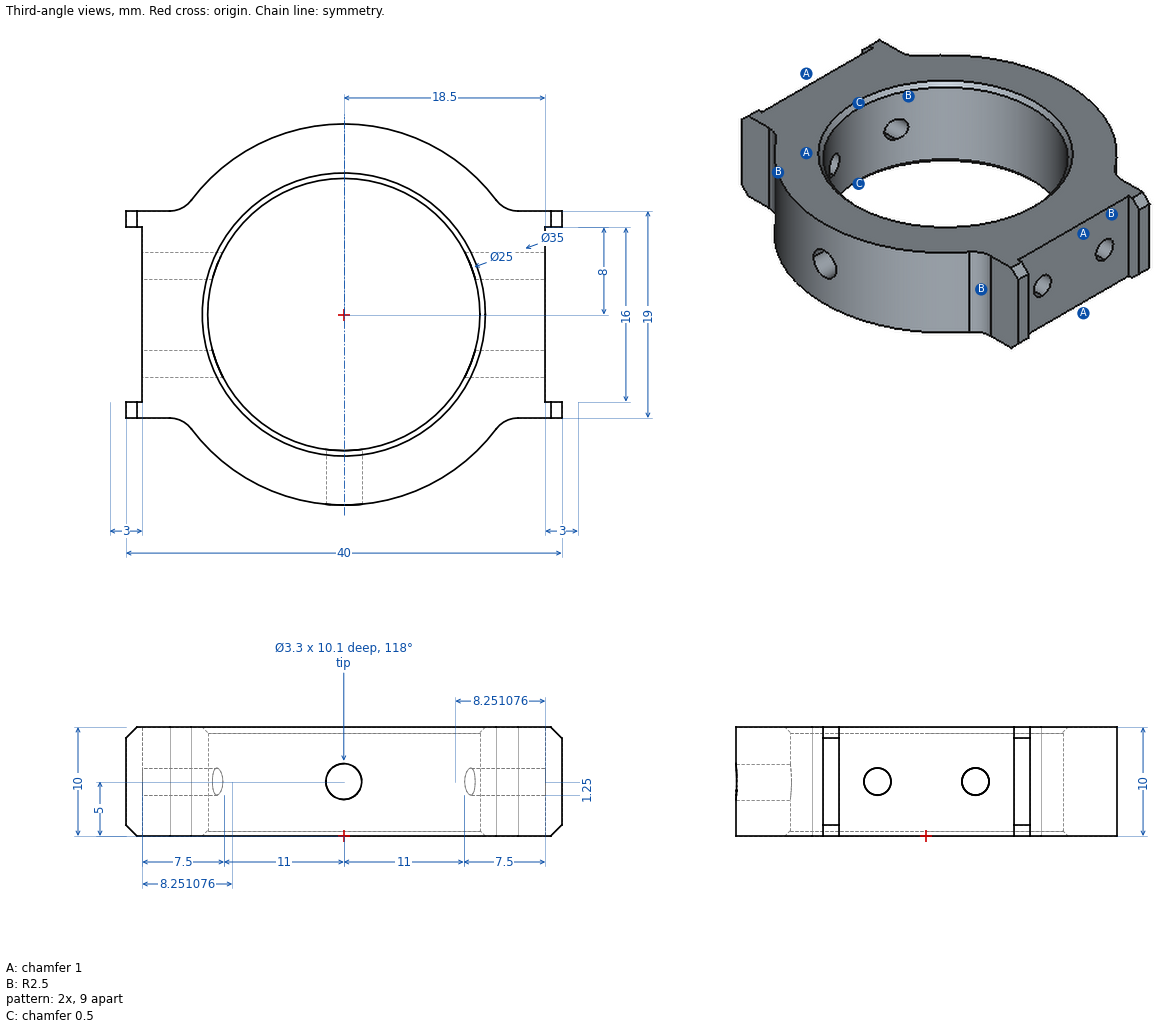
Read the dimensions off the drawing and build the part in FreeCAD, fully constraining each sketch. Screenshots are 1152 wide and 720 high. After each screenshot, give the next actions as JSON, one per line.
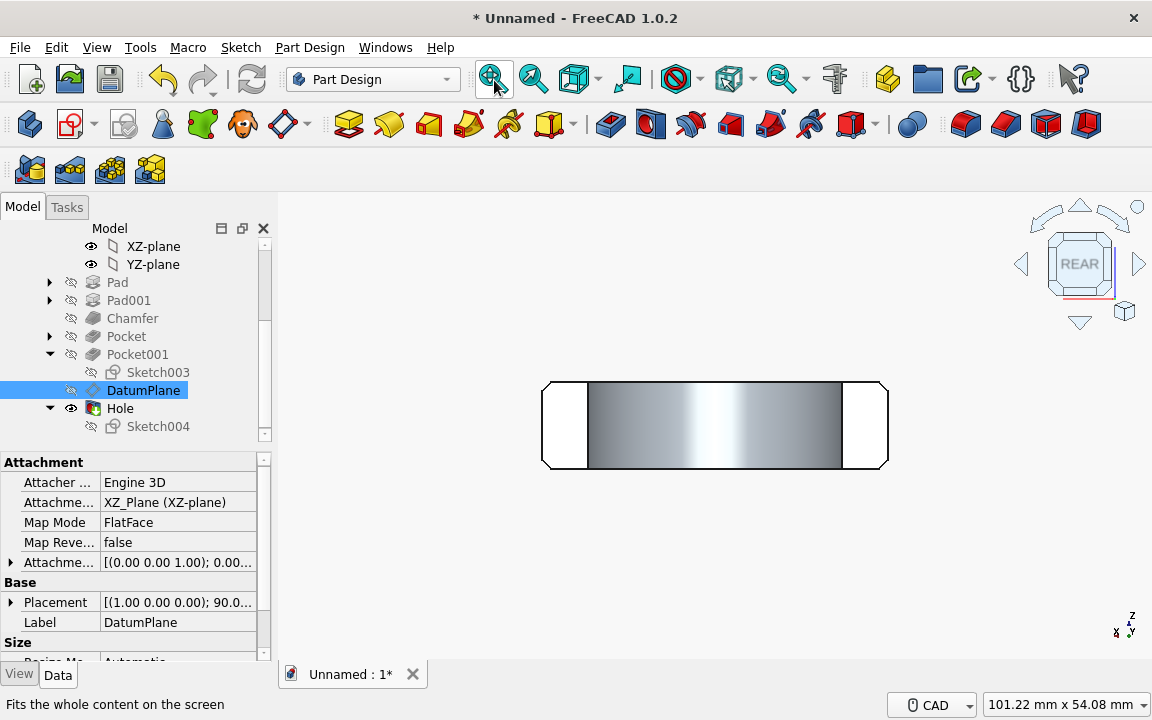
{"action": "left_click", "coordinate": [494, 80]}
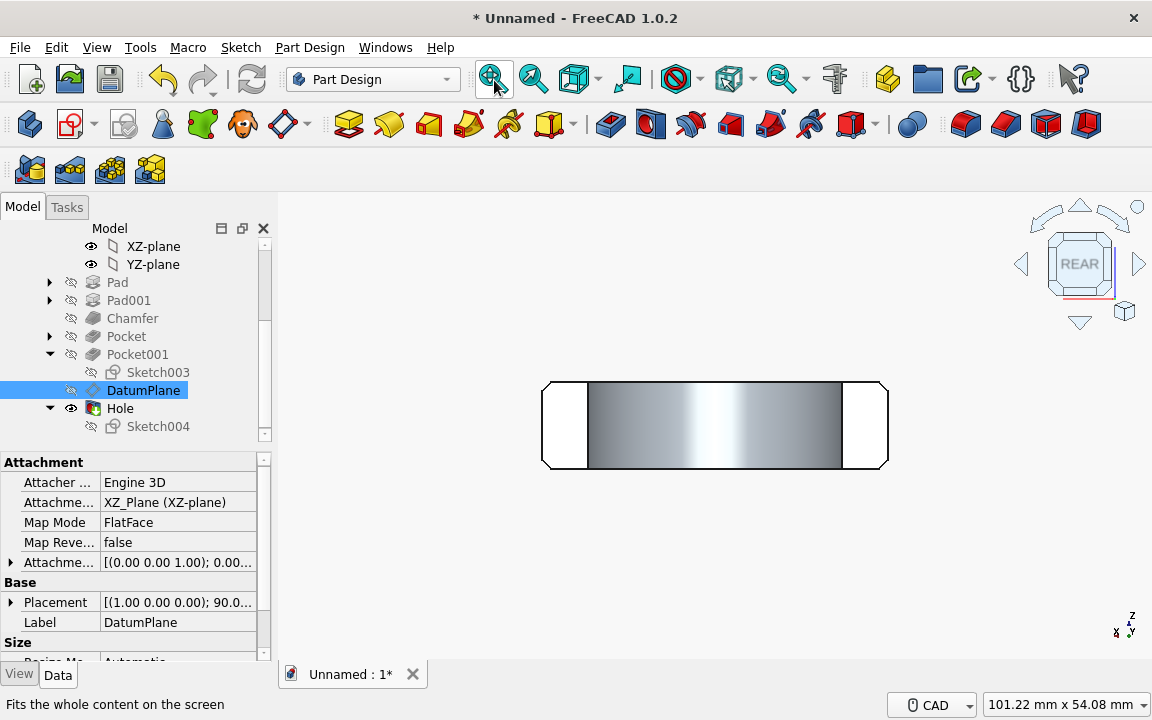
{"action": "key", "text": "6"}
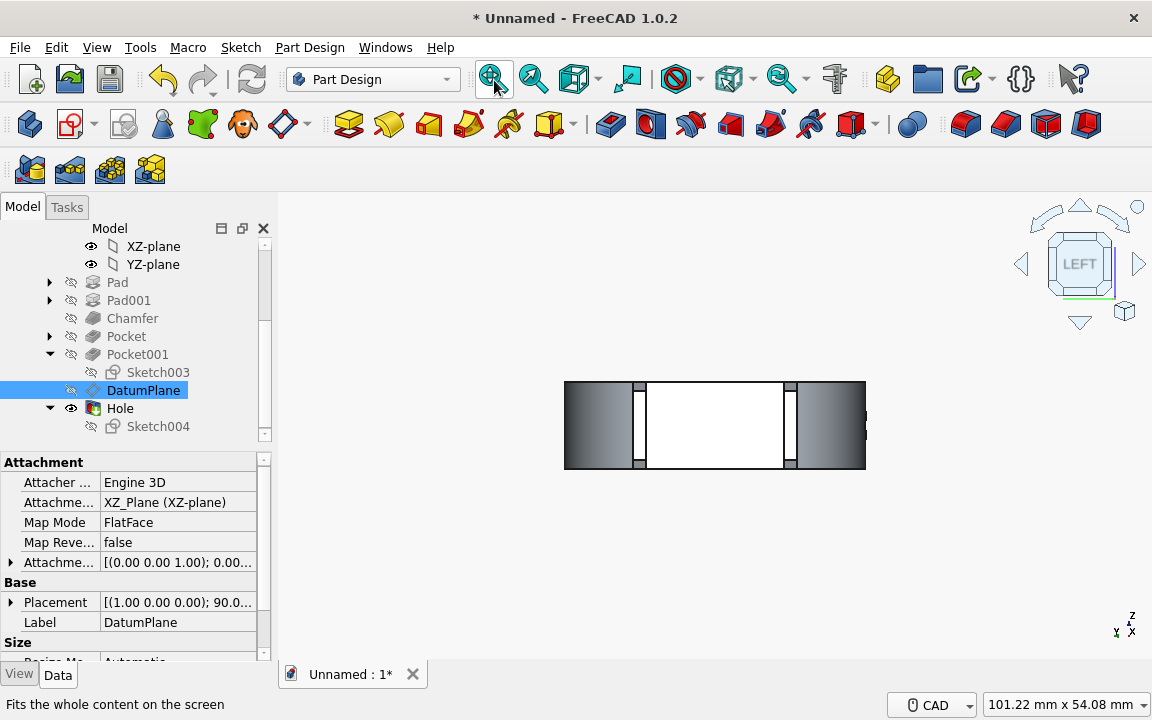
{"action": "left_click", "coordinate": [494, 80]}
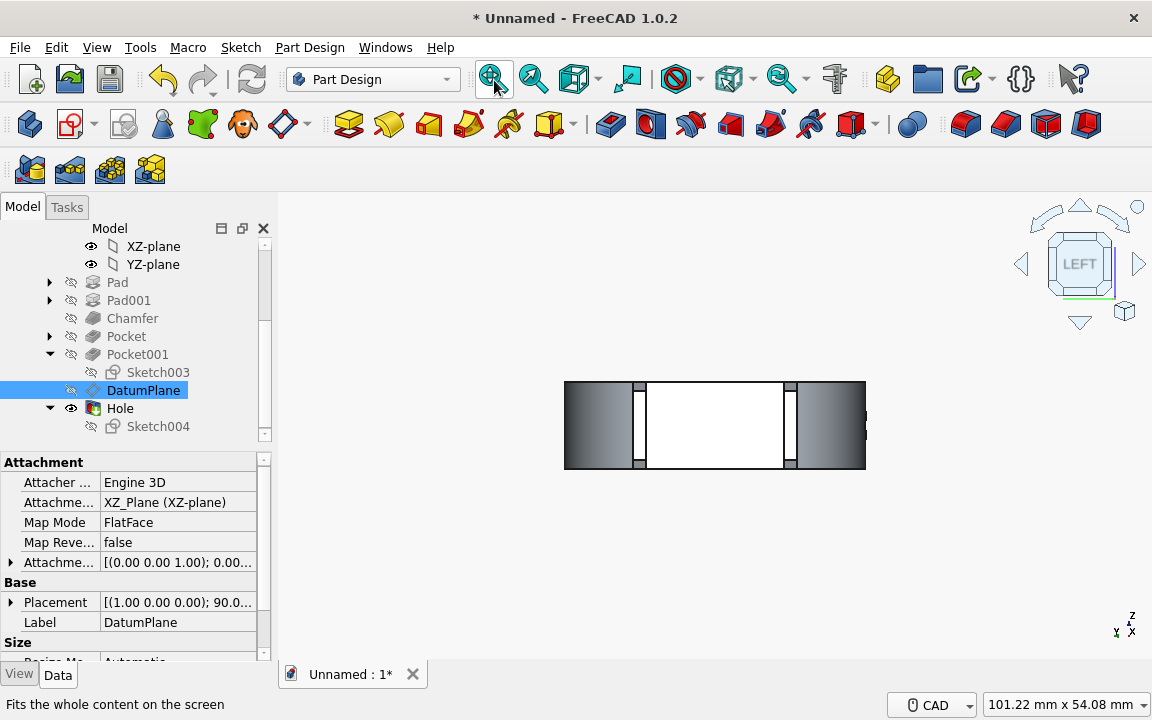
{"action": "key", "text": "v 3"}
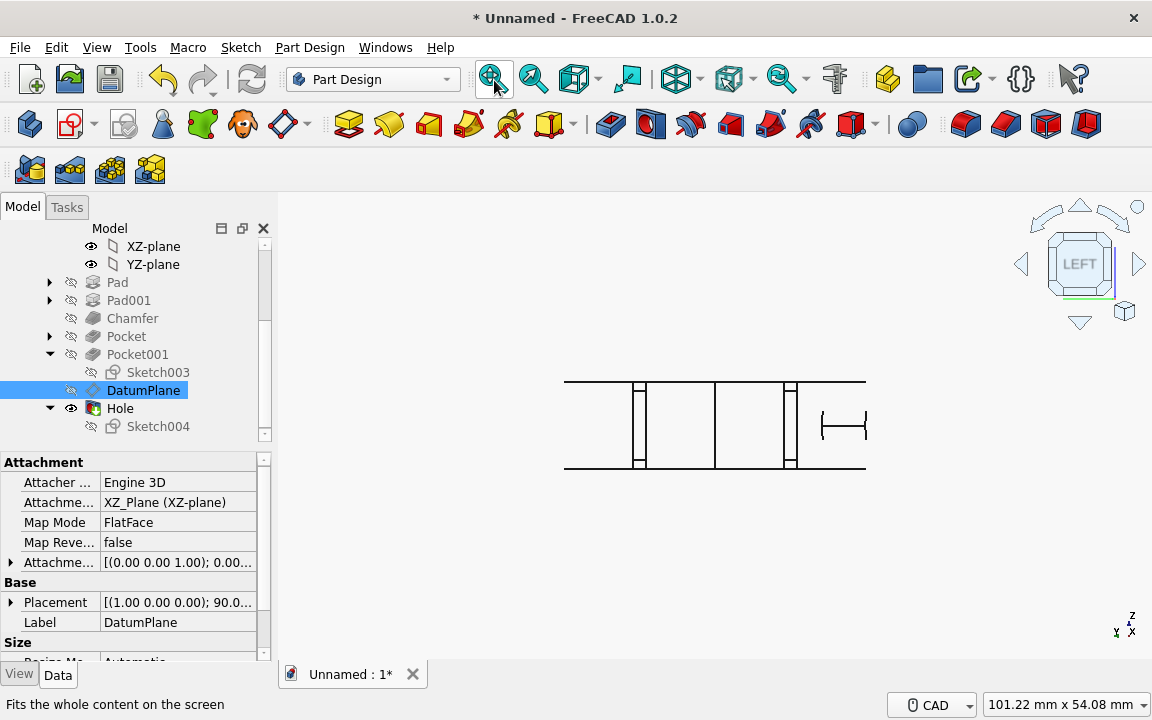
{"action": "key", "text": "0"}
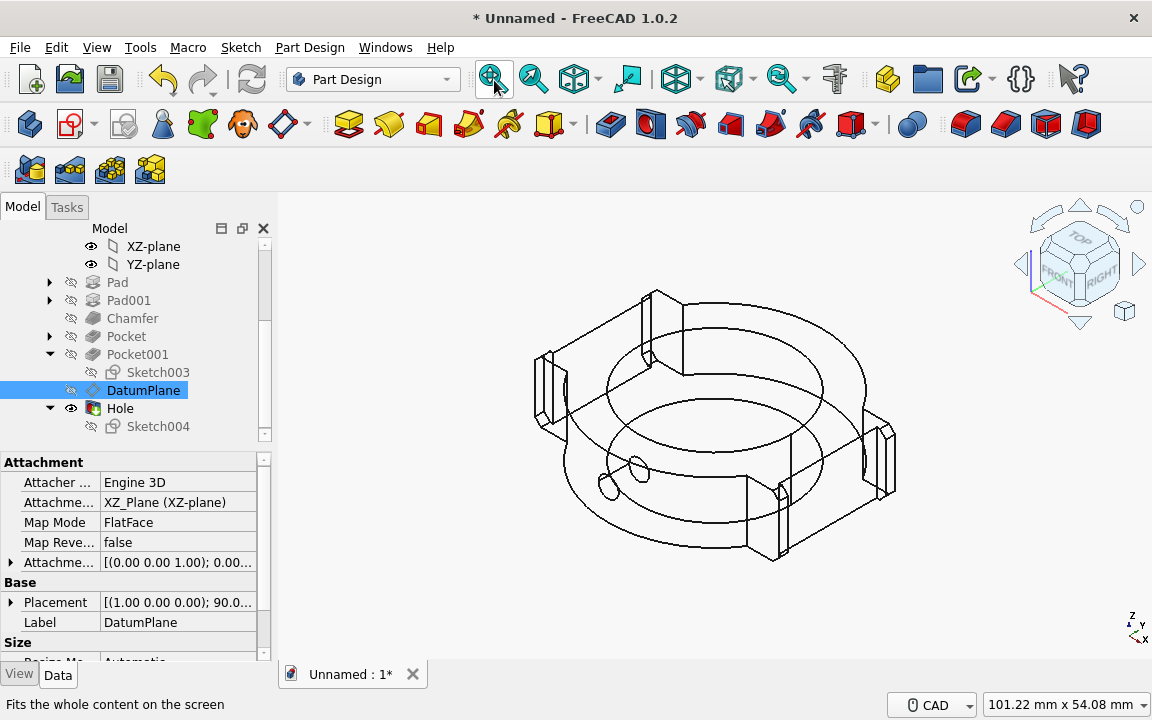
{"action": "left_click", "coordinate": [567, 427]}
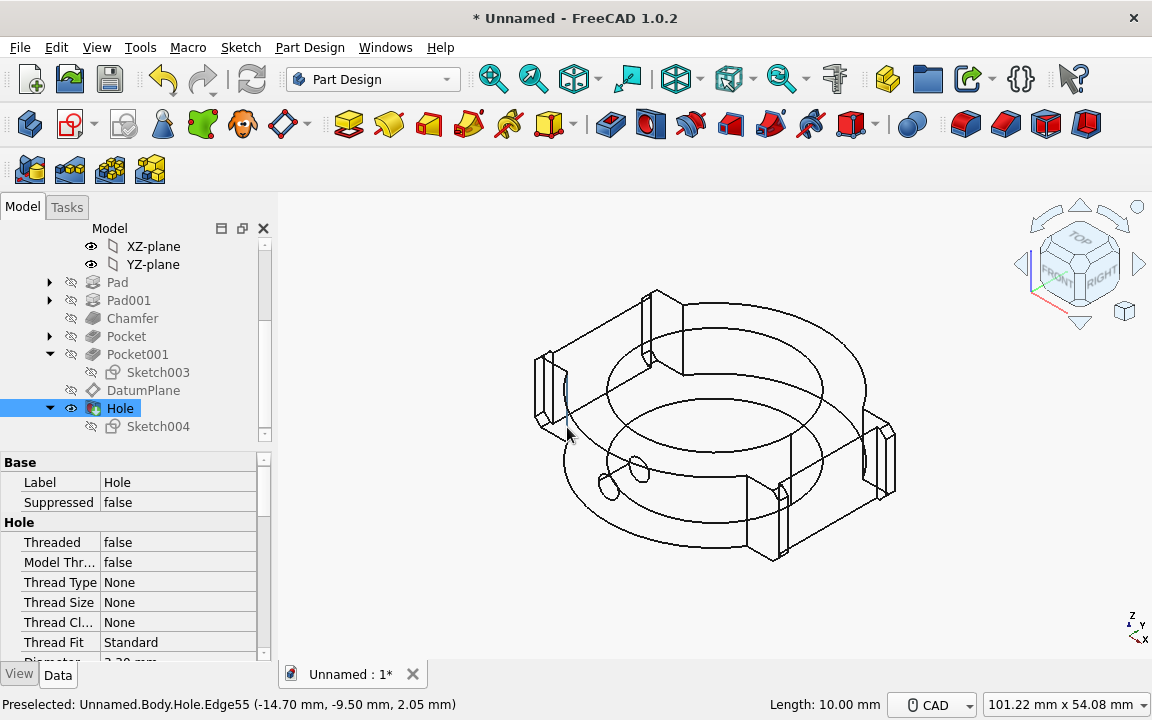
{"action": "left_click", "coordinate": [747, 510], "text": "ctrl"}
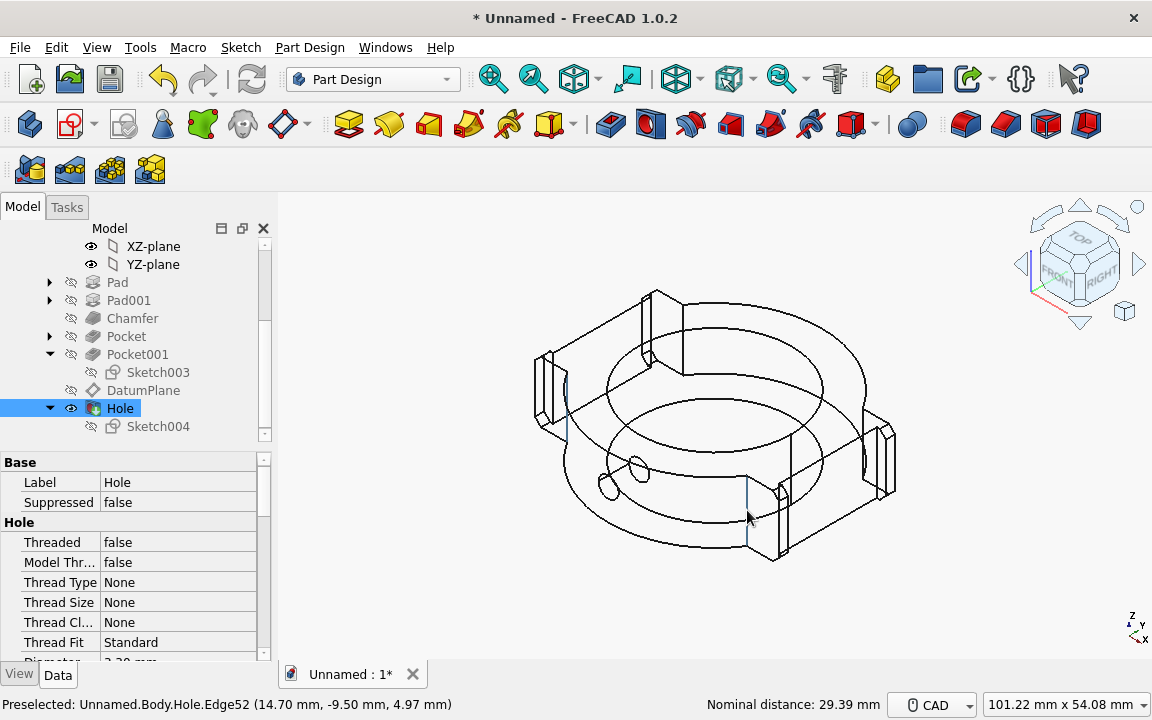
{"action": "left_click", "coordinate": [863, 443], "text": "ctrl"}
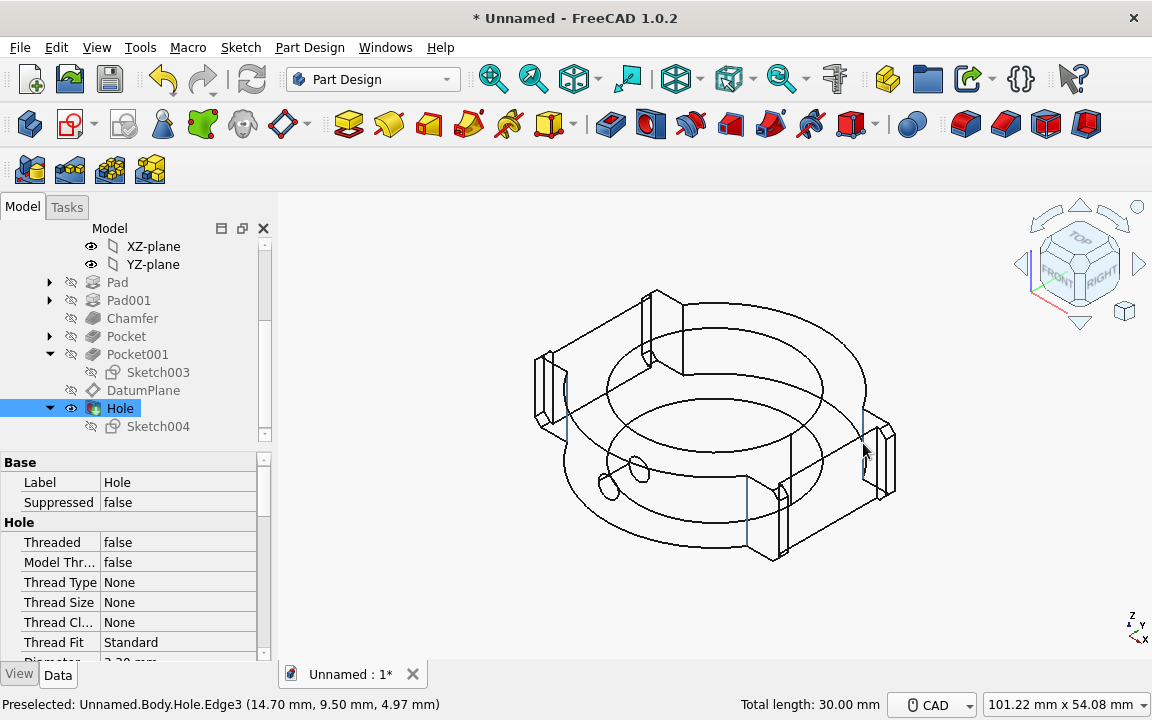
{"action": "left_click", "coordinate": [683, 339], "text": "ctrl"}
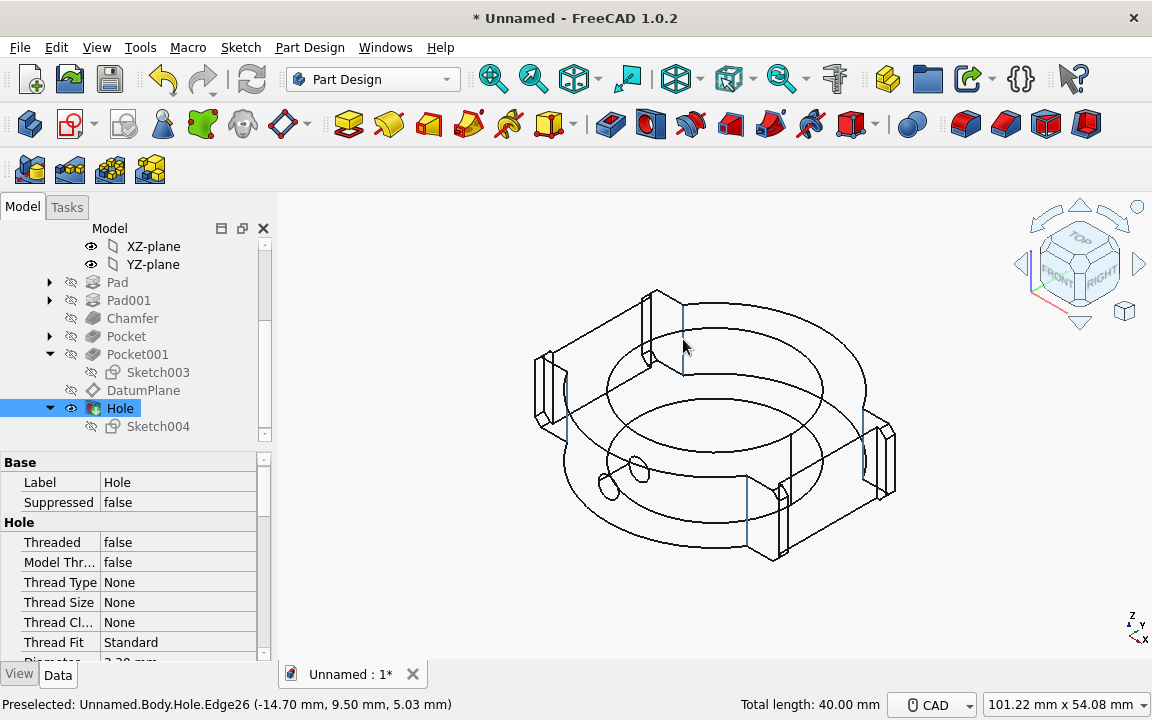
{"action": "key", "text": "v 1"}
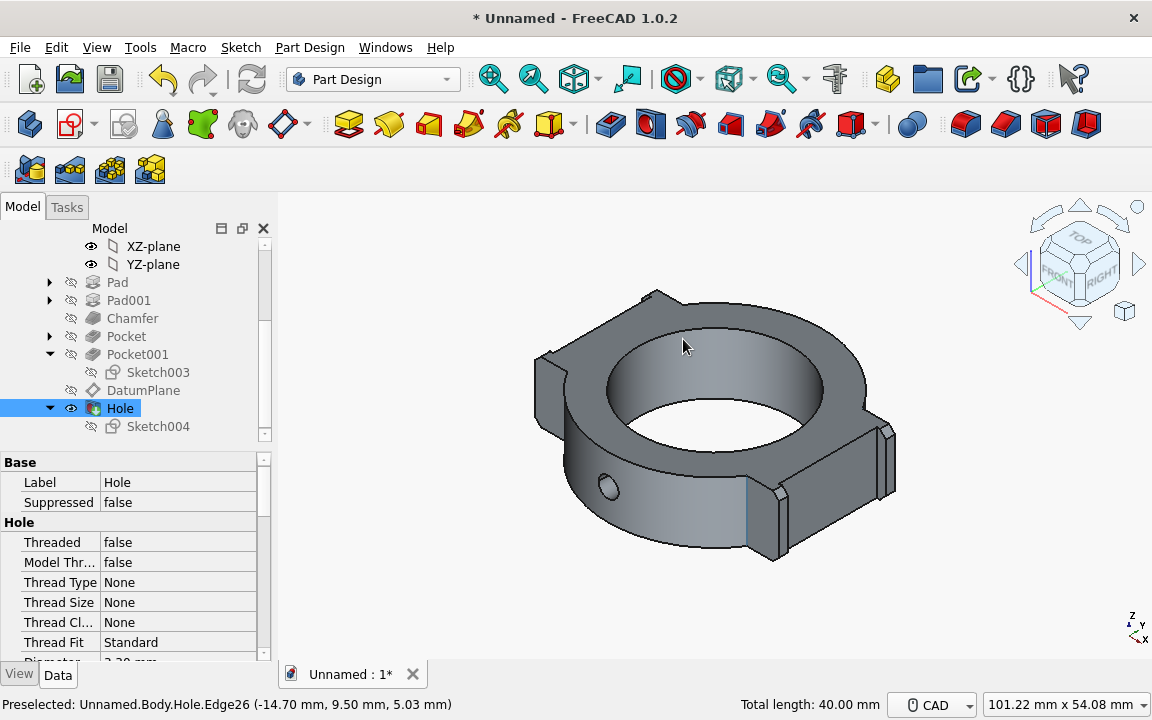
{"action": "left_click", "coordinate": [966, 124]}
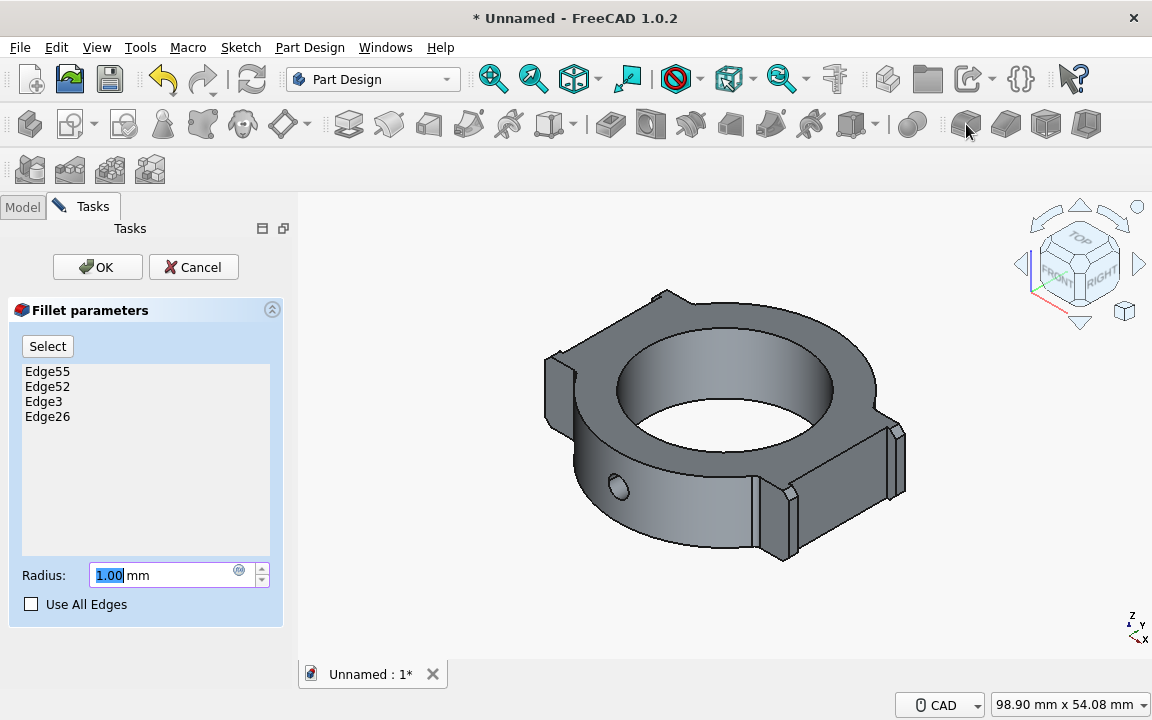
{"action": "type", "text": "2.5"}
{"action": "key", "text": "Tab"}